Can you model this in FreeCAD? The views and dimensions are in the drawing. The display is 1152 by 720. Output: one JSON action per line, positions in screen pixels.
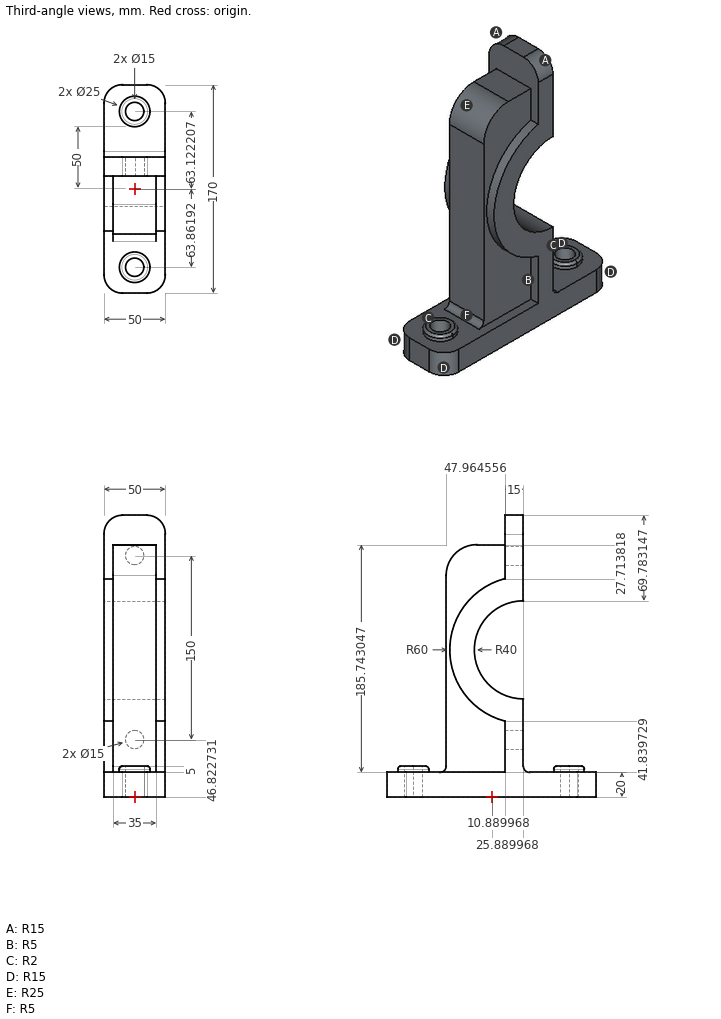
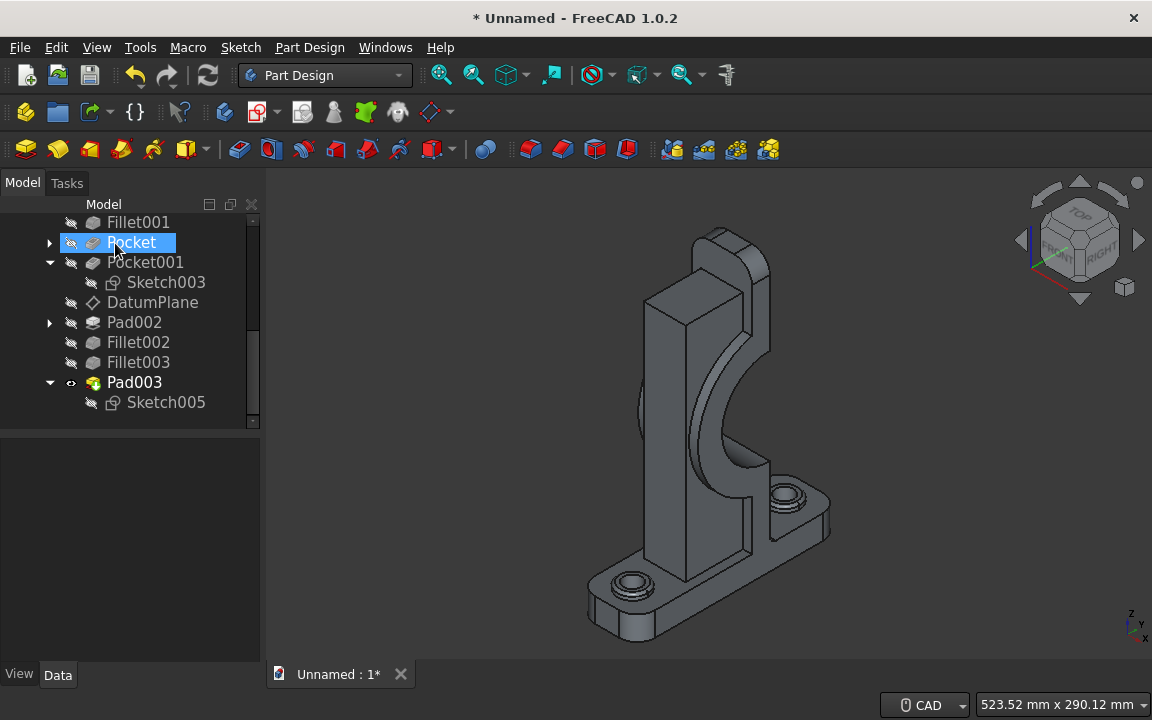
{"action": "left_click", "coordinate": [665, 313]}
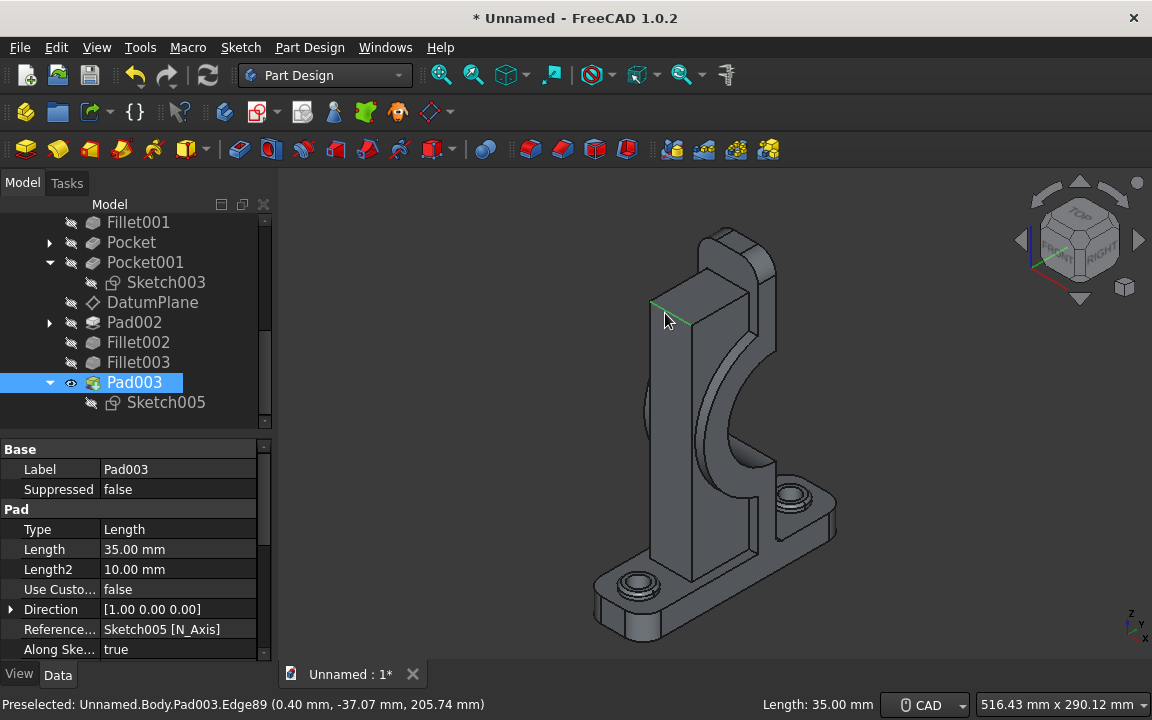
{"action": "left_click", "coordinate": [532, 150]}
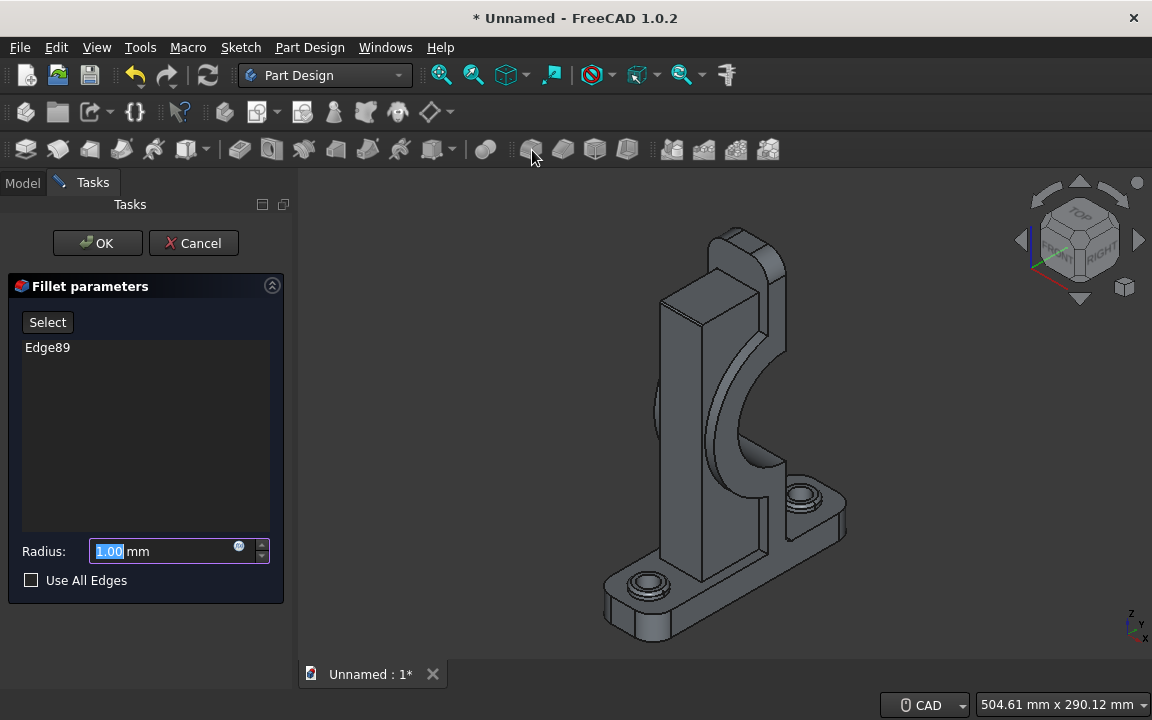
{"action": "type", "text": "25"}
{"action": "key", "text": "Tab"}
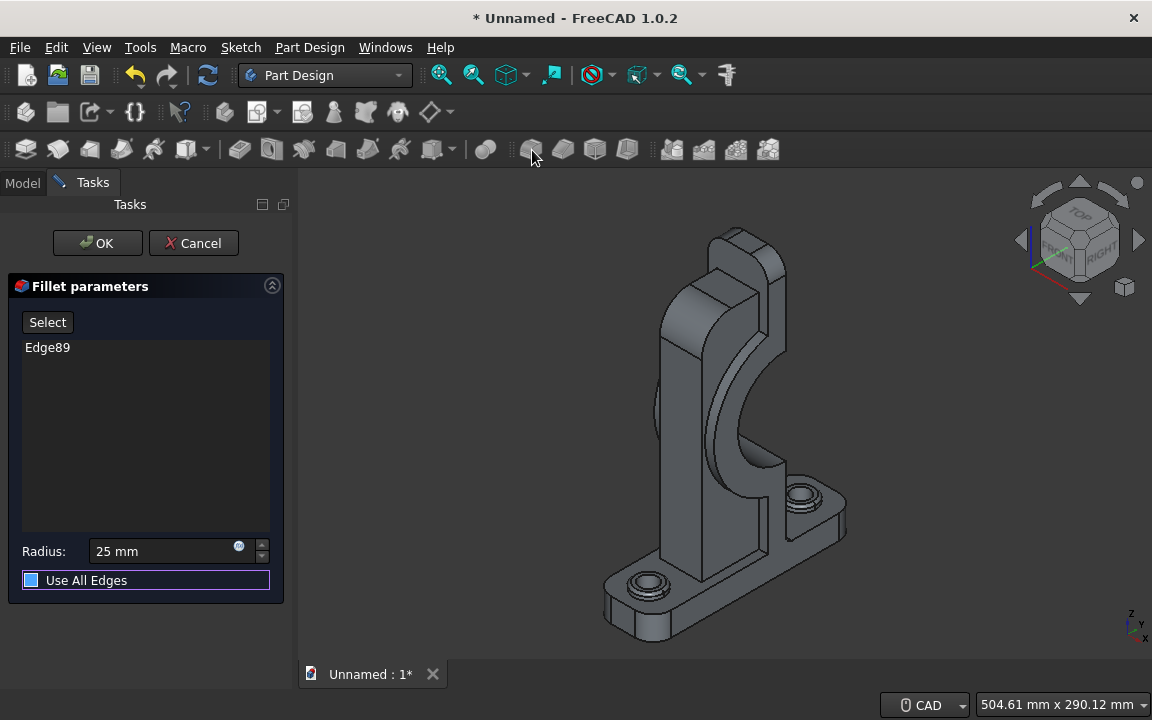
{"action": "left_click", "coordinate": [98, 243]}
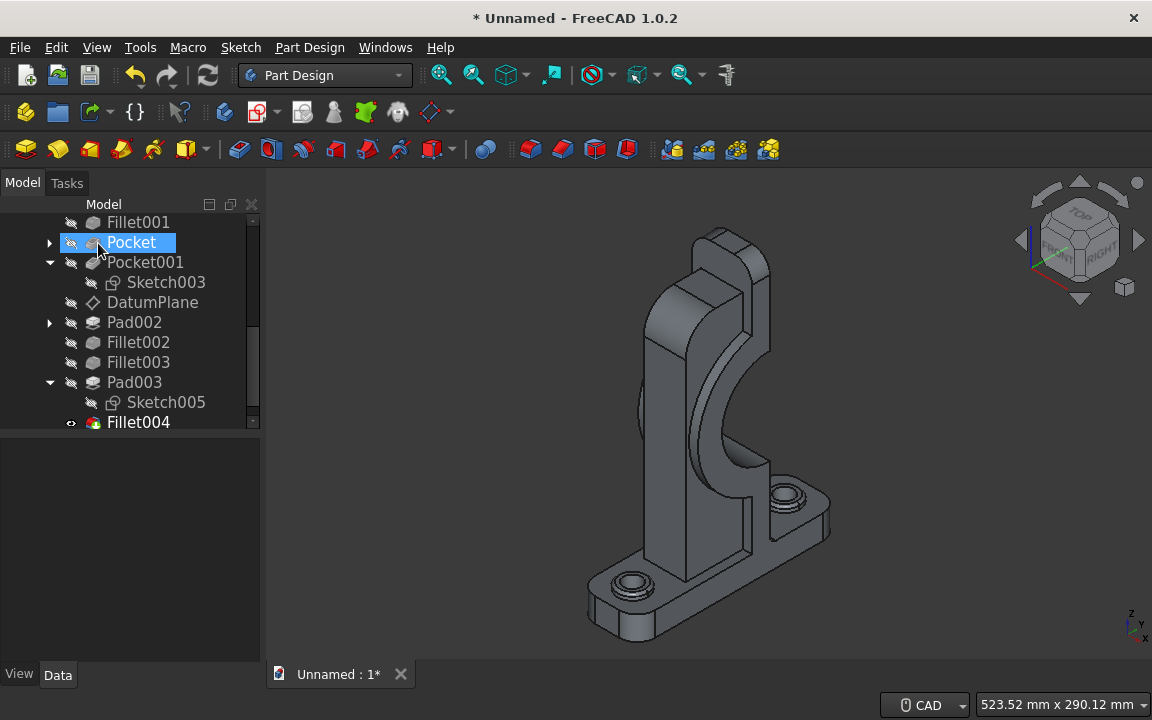
{"action": "key", "text": "2"}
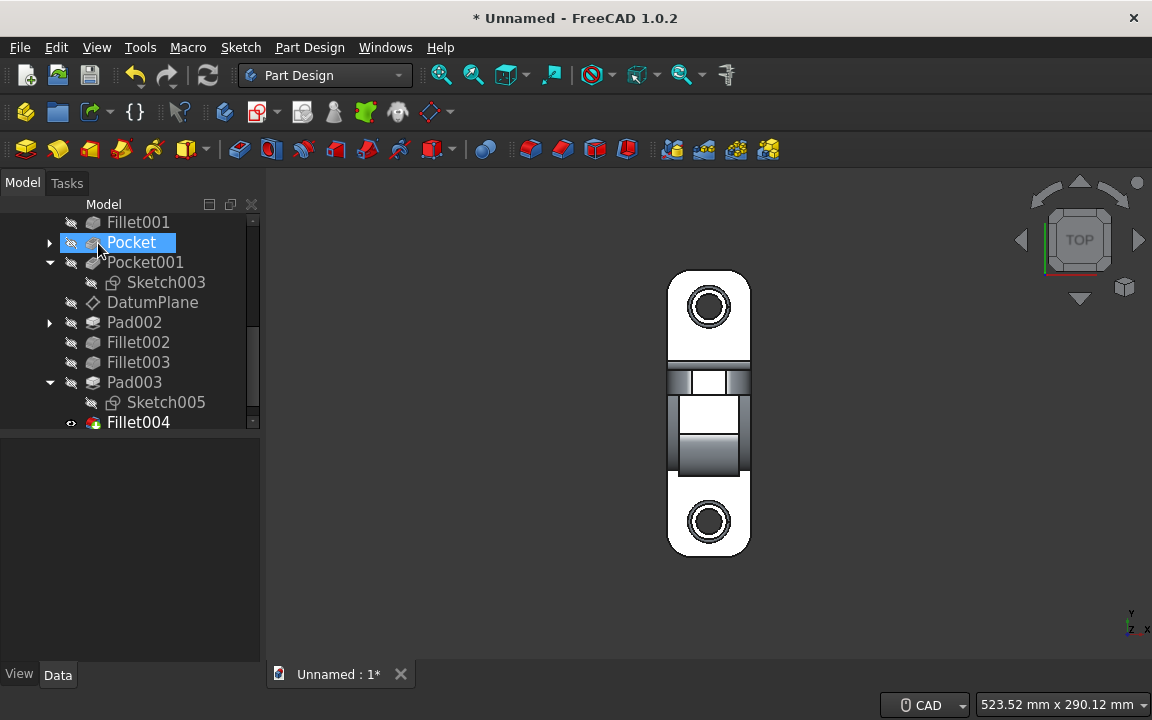
{"action": "key", "text": "0"}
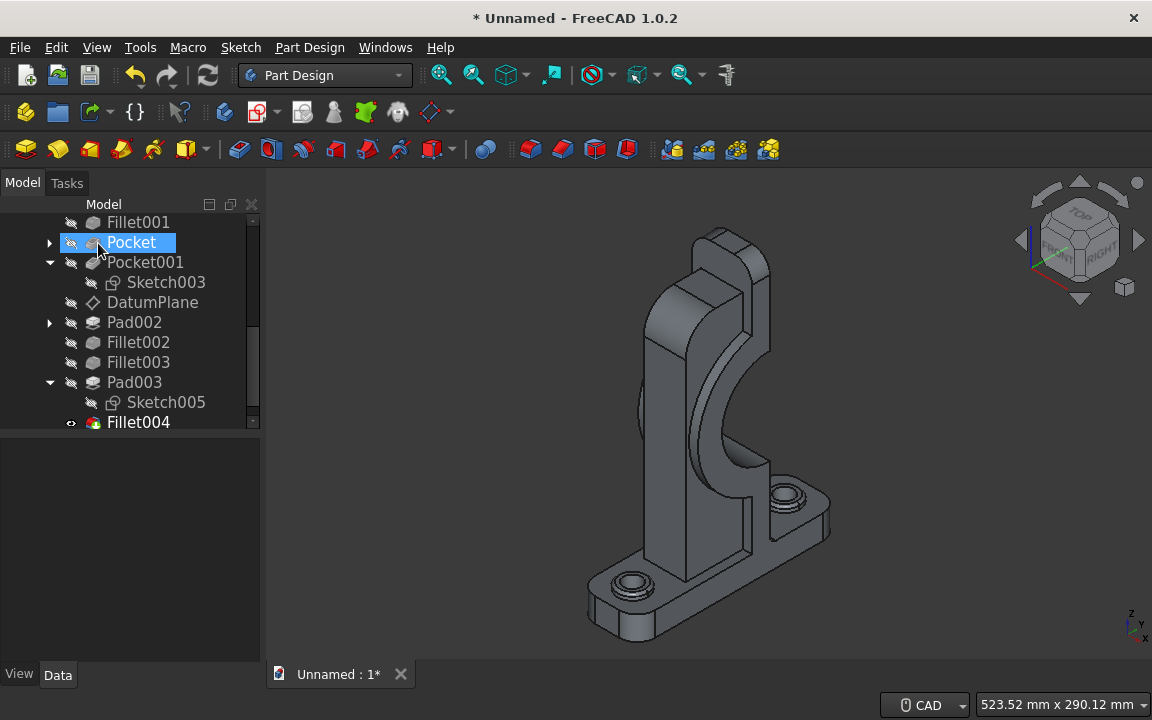
{"action": "key", "text": "1"}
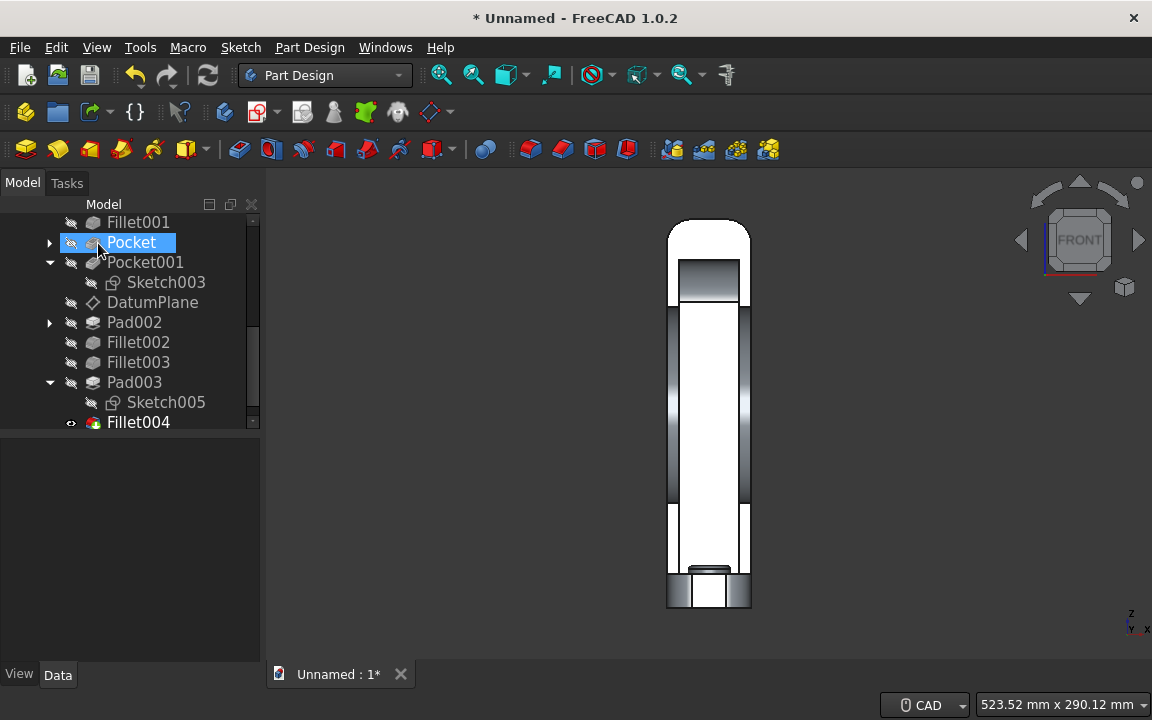
{"action": "key", "text": "3"}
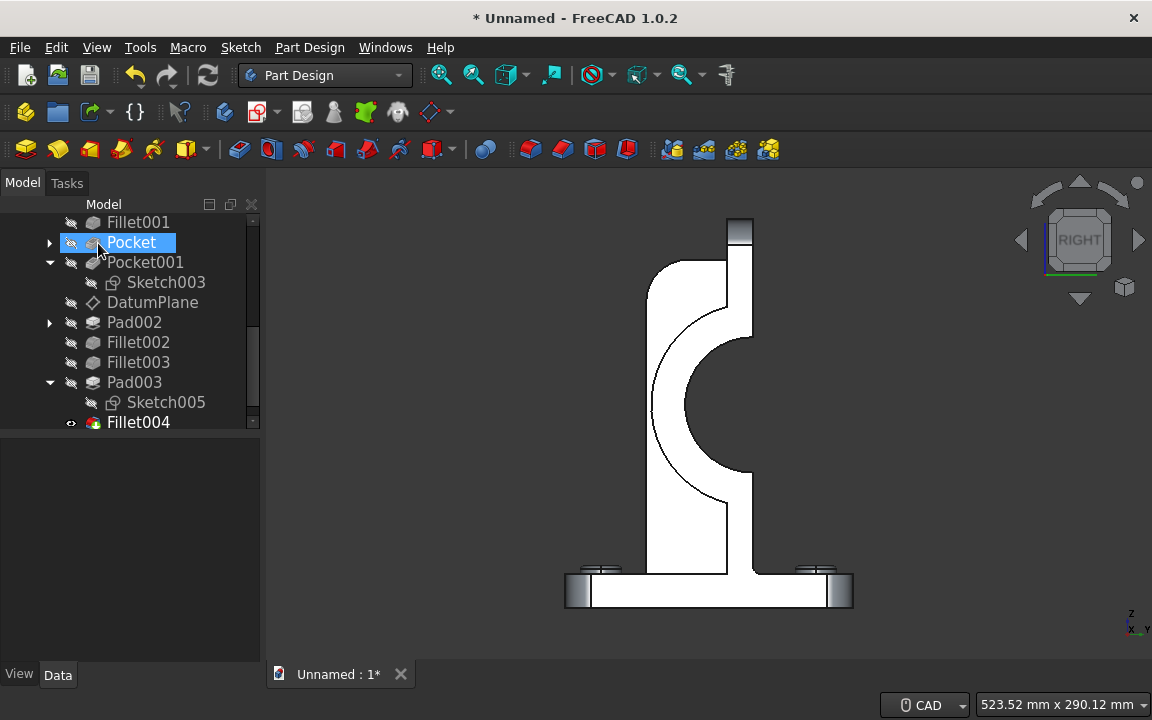
{"action": "key", "text": "5"}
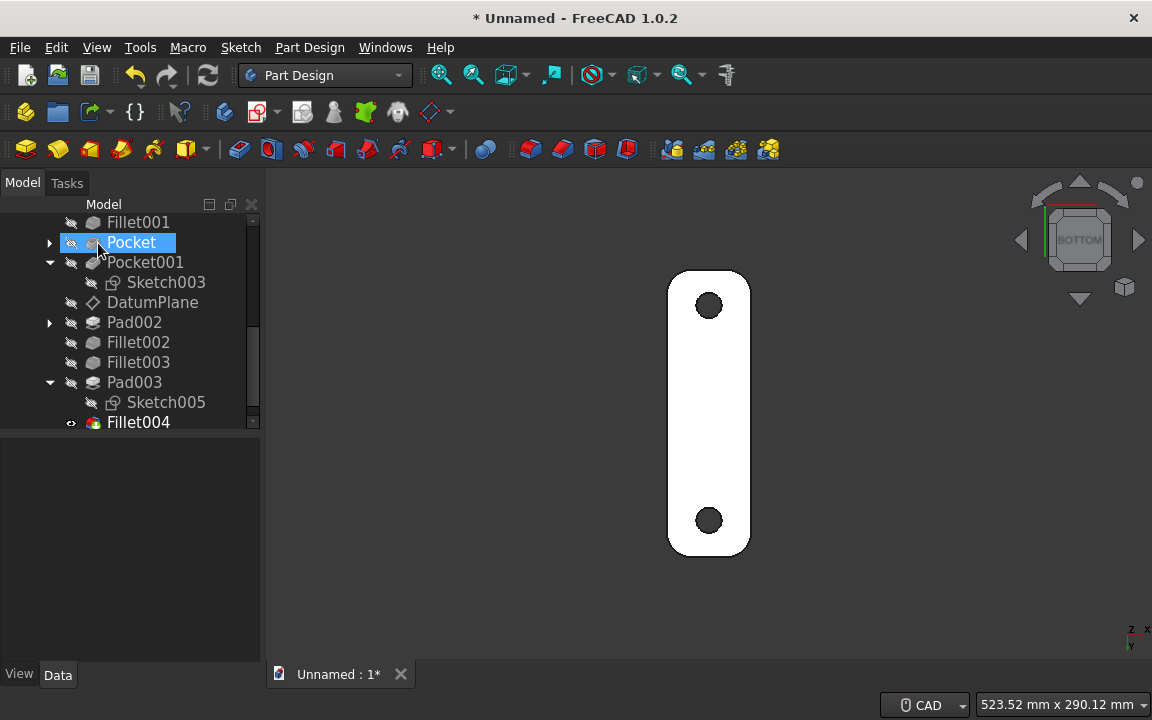
{"action": "key", "text": "4"}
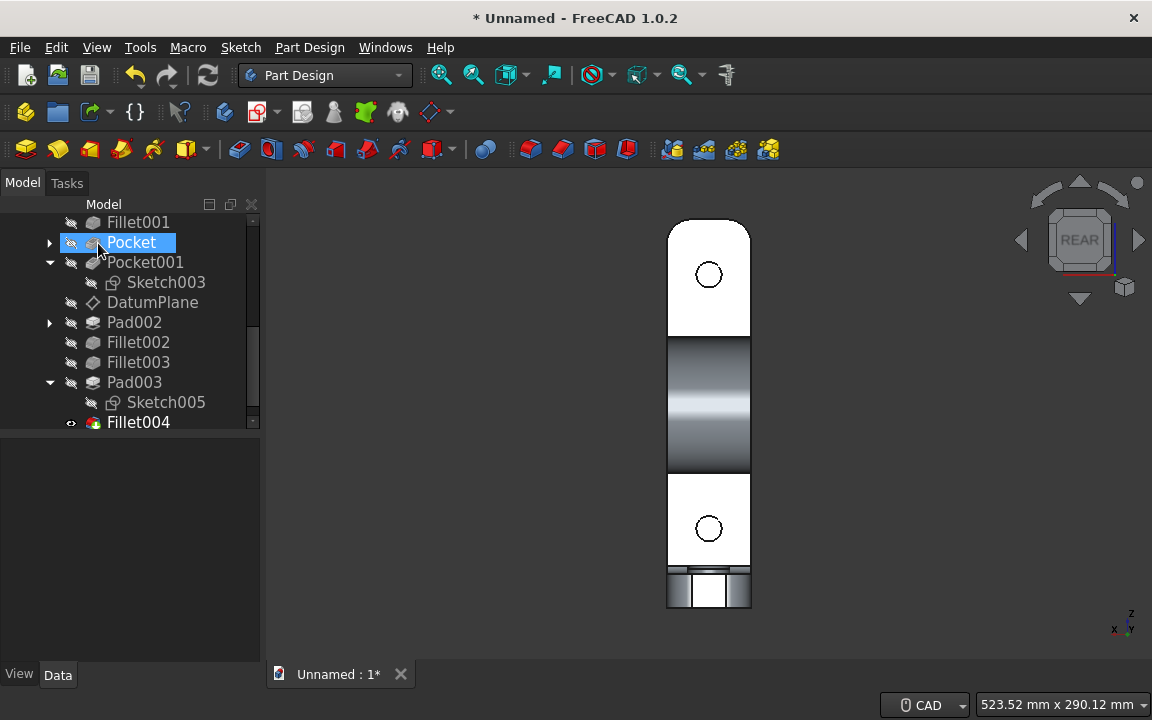
{"action": "key", "text": "6"}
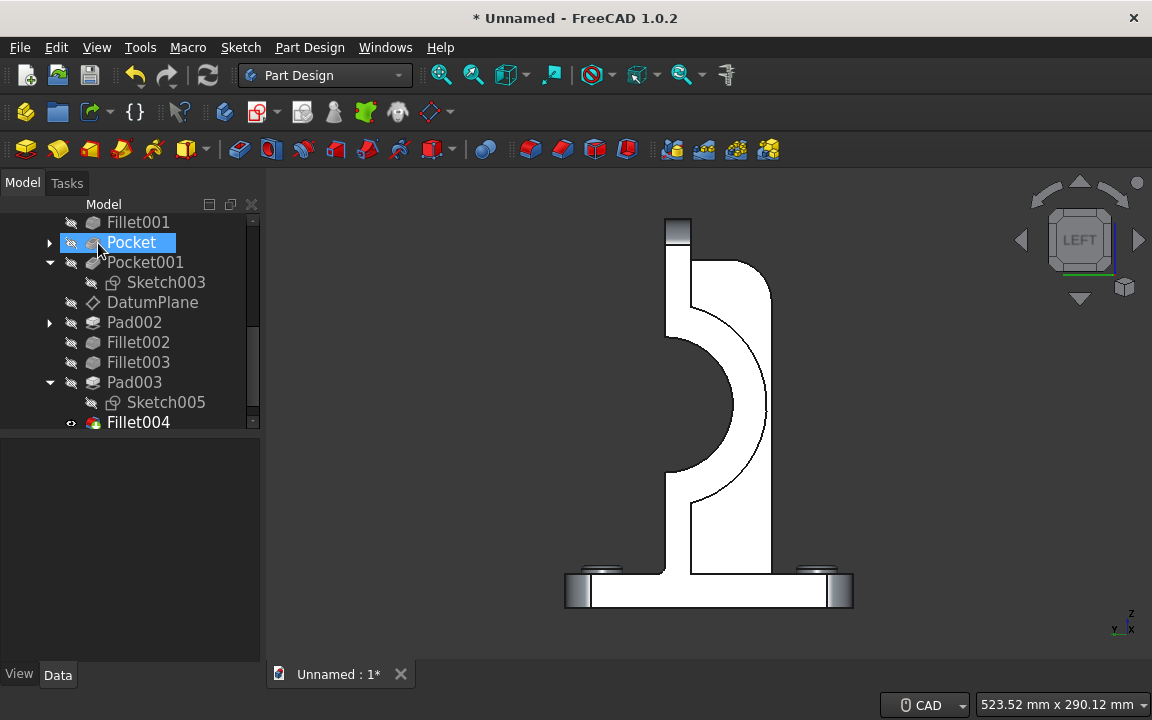
{"action": "key", "text": "v 3"}